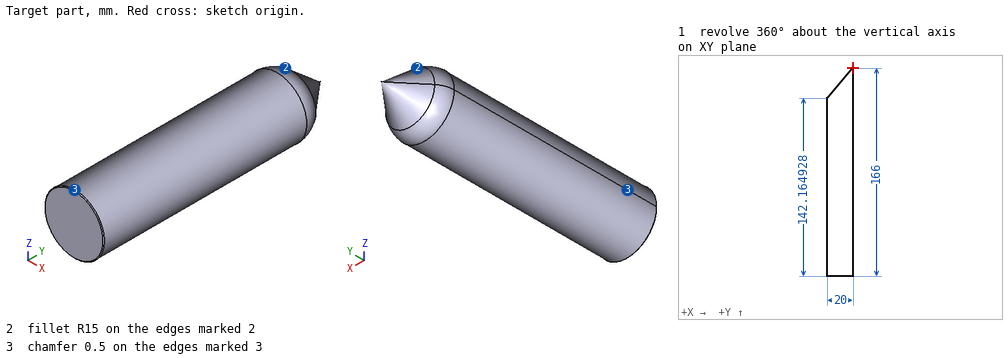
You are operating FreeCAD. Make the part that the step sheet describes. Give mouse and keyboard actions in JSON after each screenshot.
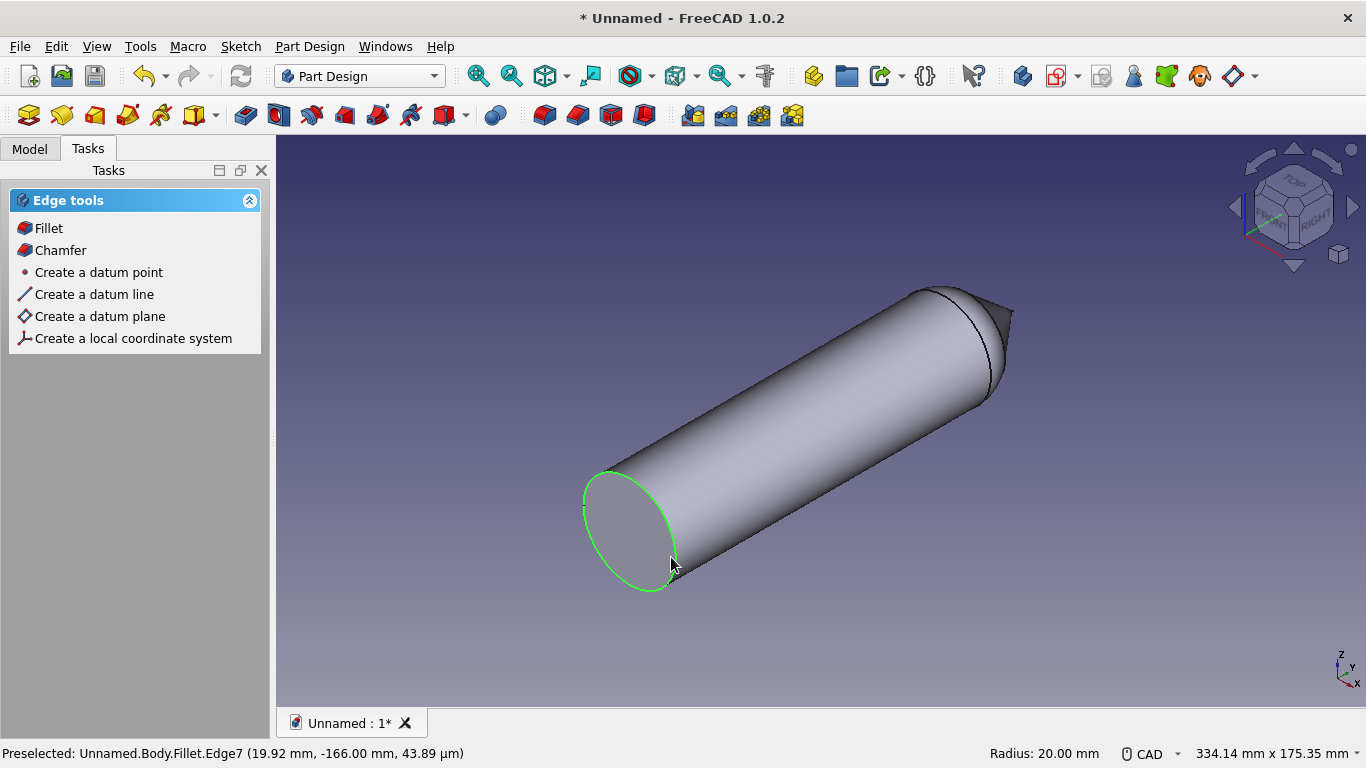
{"action": "left_click", "coordinate": [578, 116]}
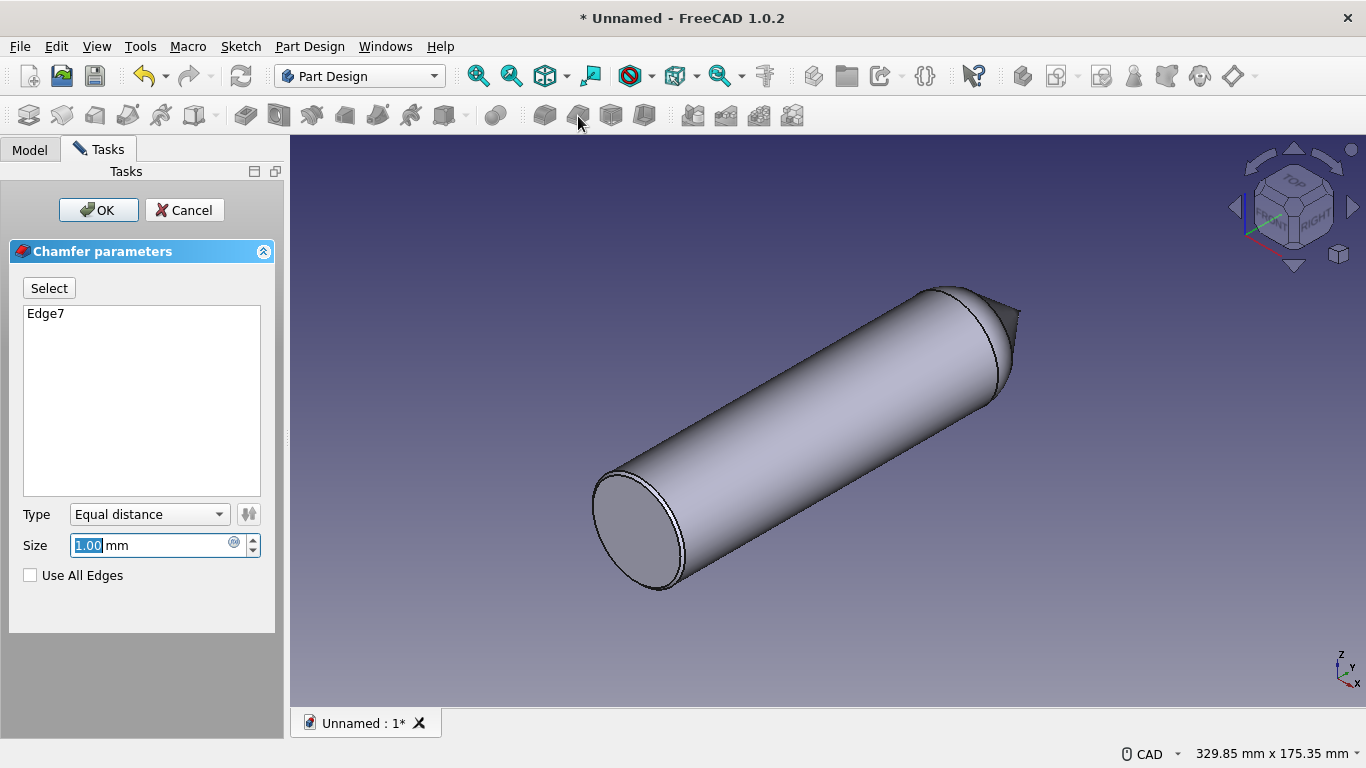
{"action": "type", "text": "0.5"}
{"action": "key", "text": "Tab"}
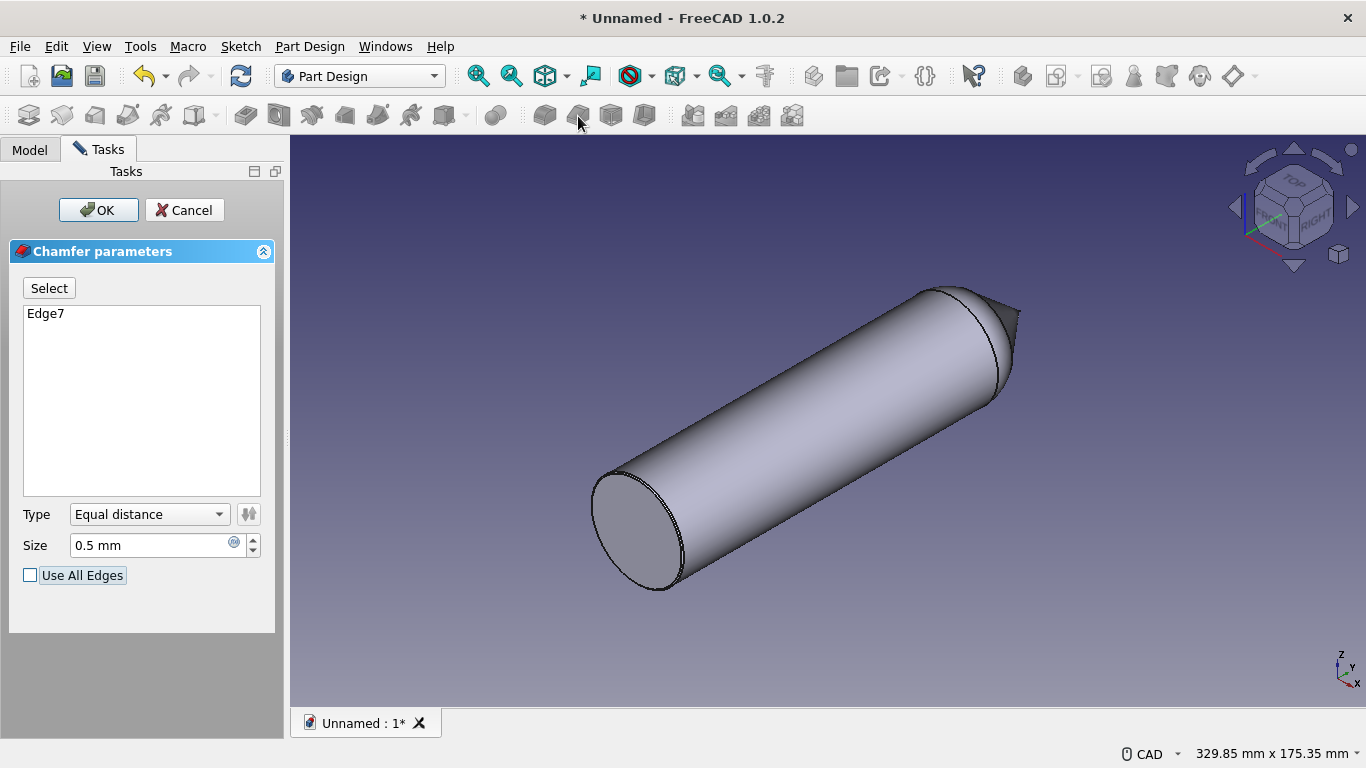
{"action": "left_click", "coordinate": [99, 210]}